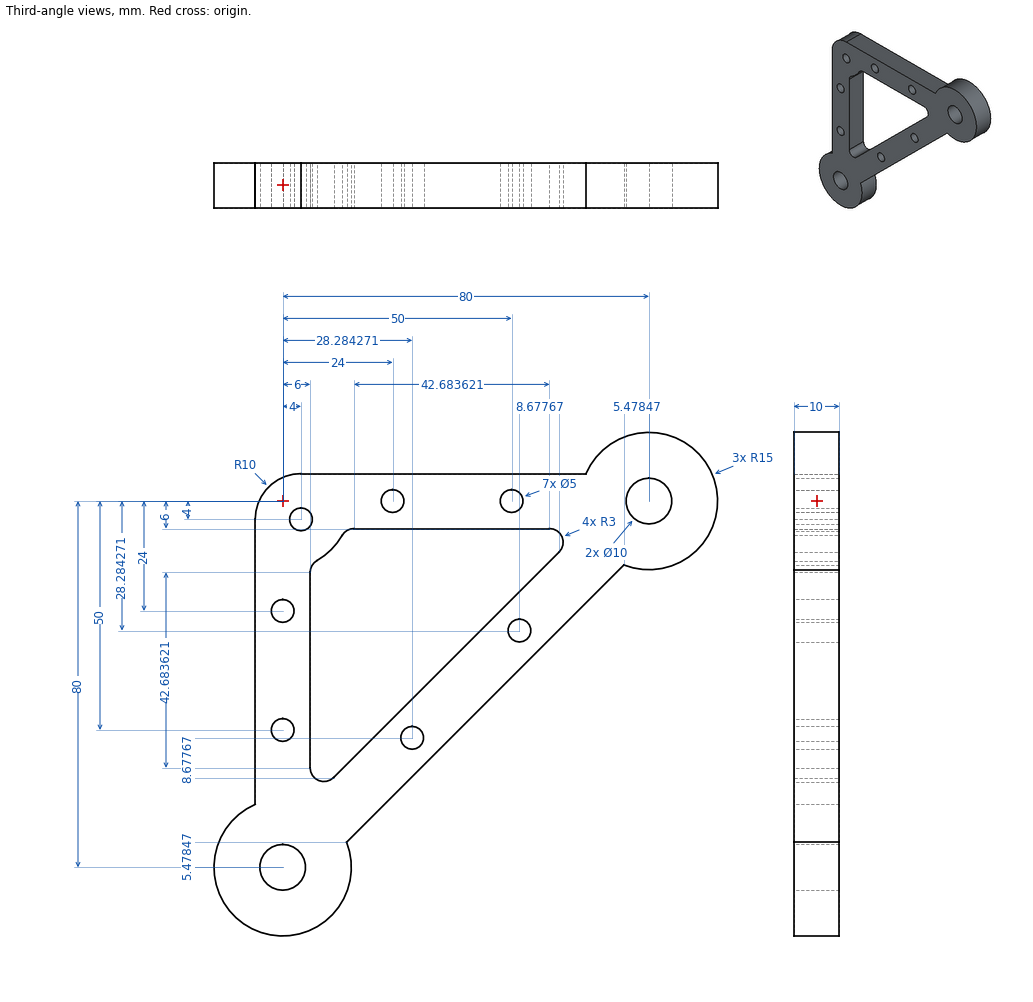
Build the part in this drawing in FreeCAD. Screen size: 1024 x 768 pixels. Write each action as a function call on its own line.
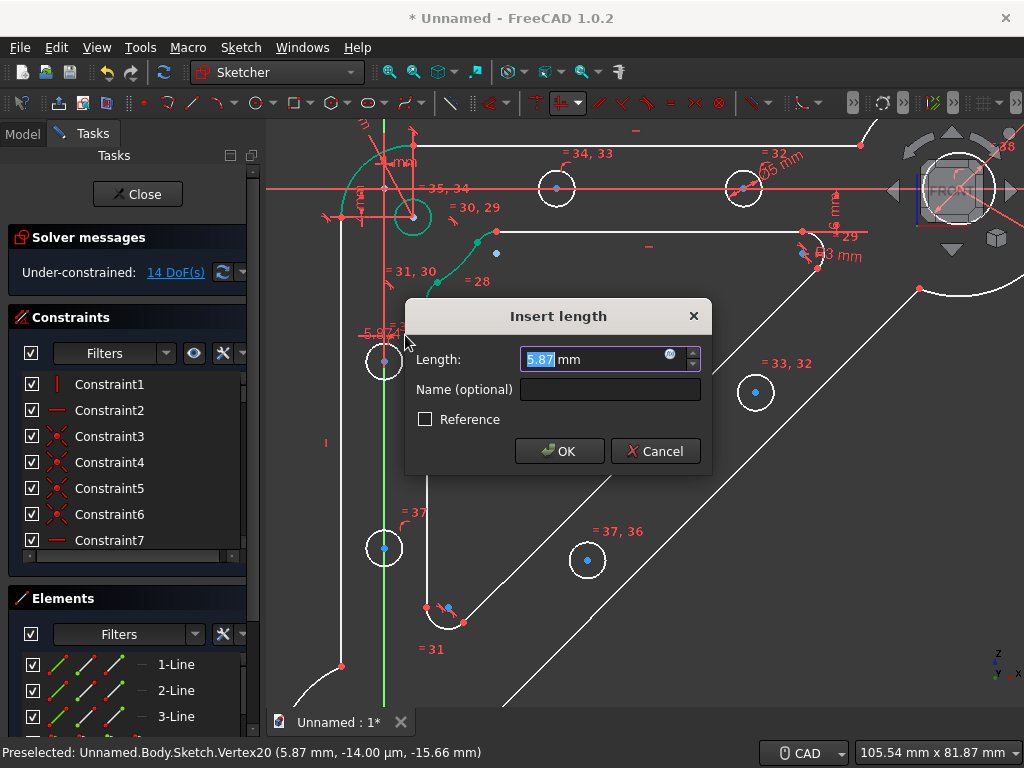
text(6)
key(Return)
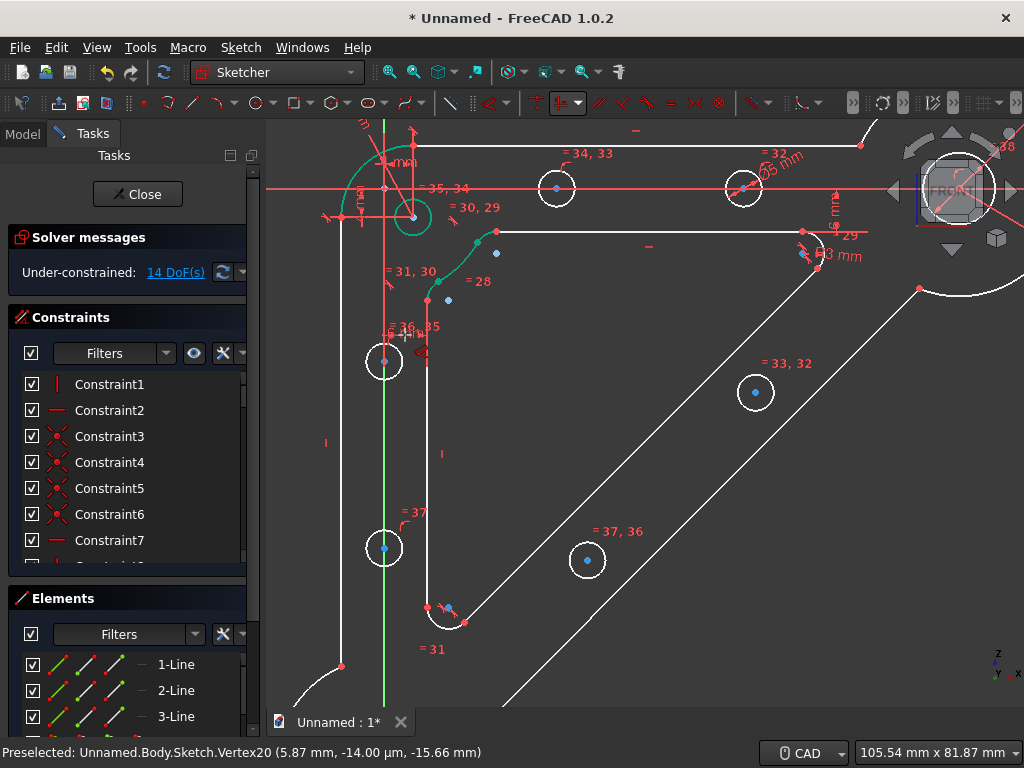
scroll(426, 302, down, 3)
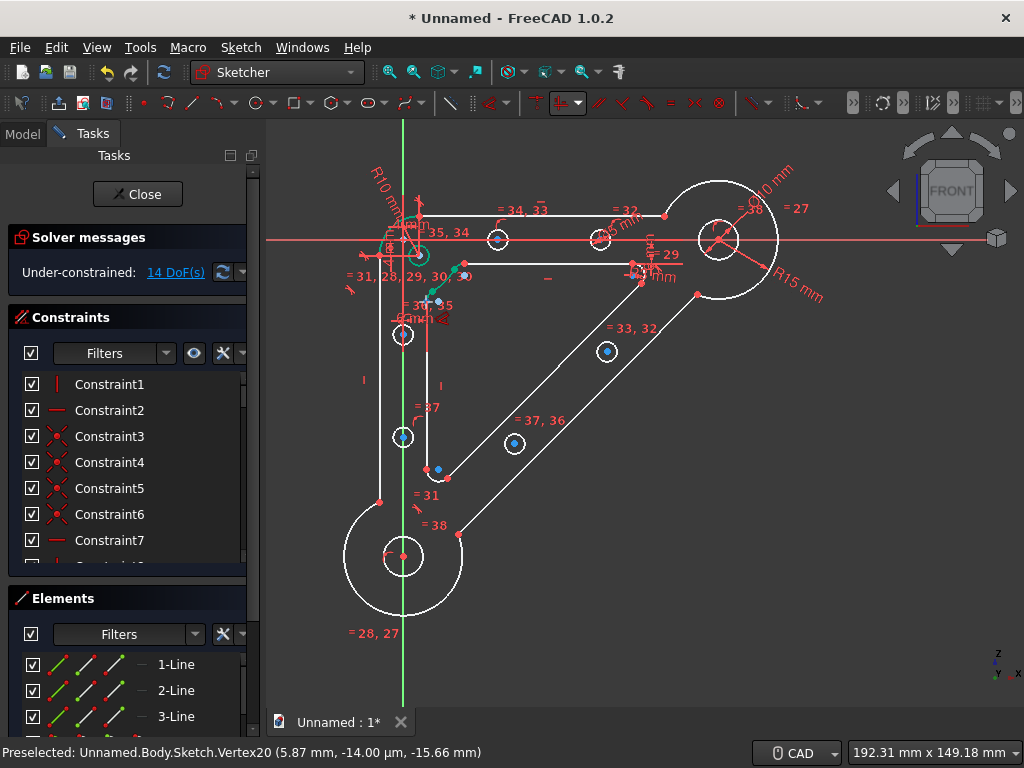
click(719, 240)
click(561, 182)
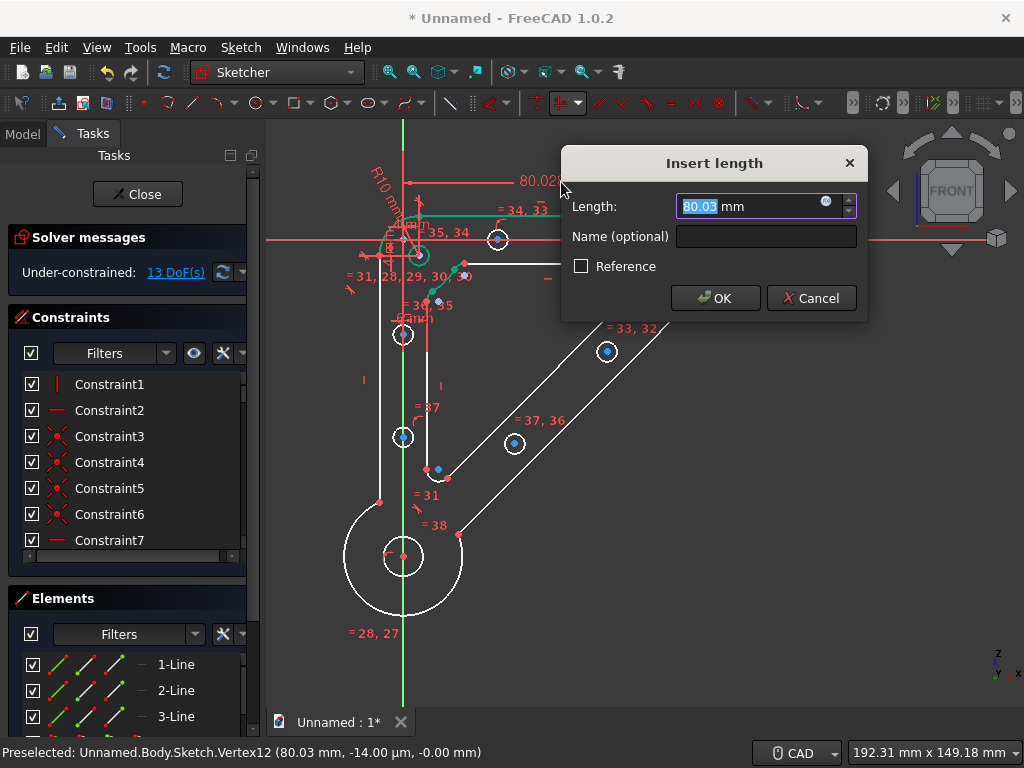
text(80)
key(Return)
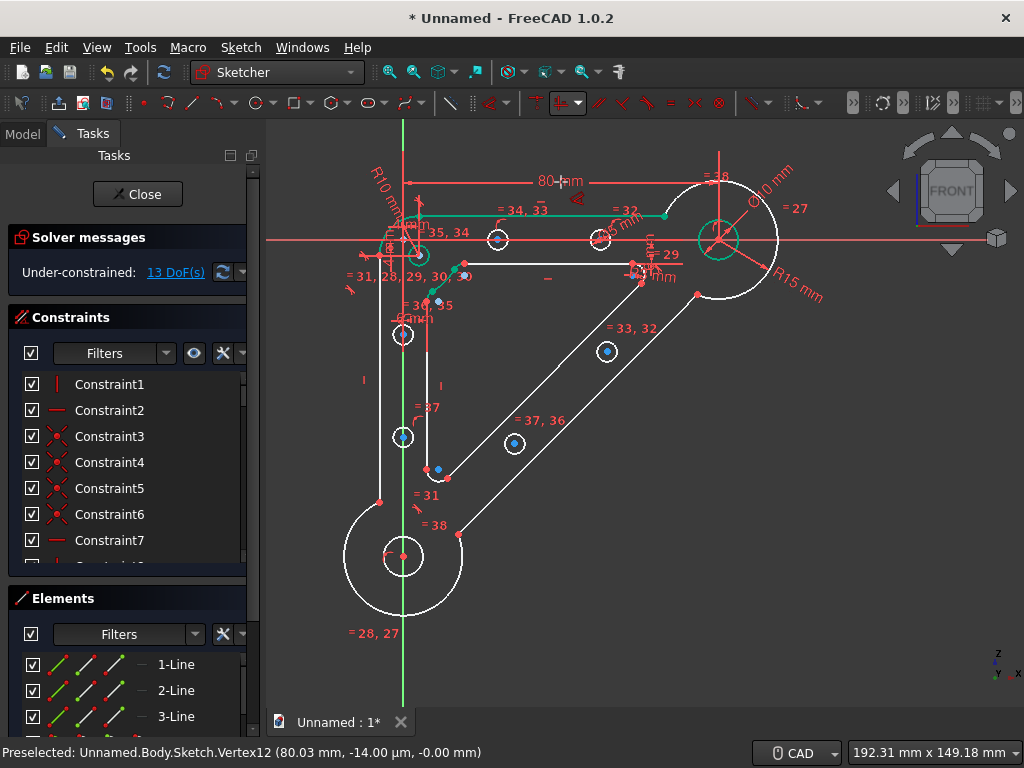
click(600, 240)
click(433, 274)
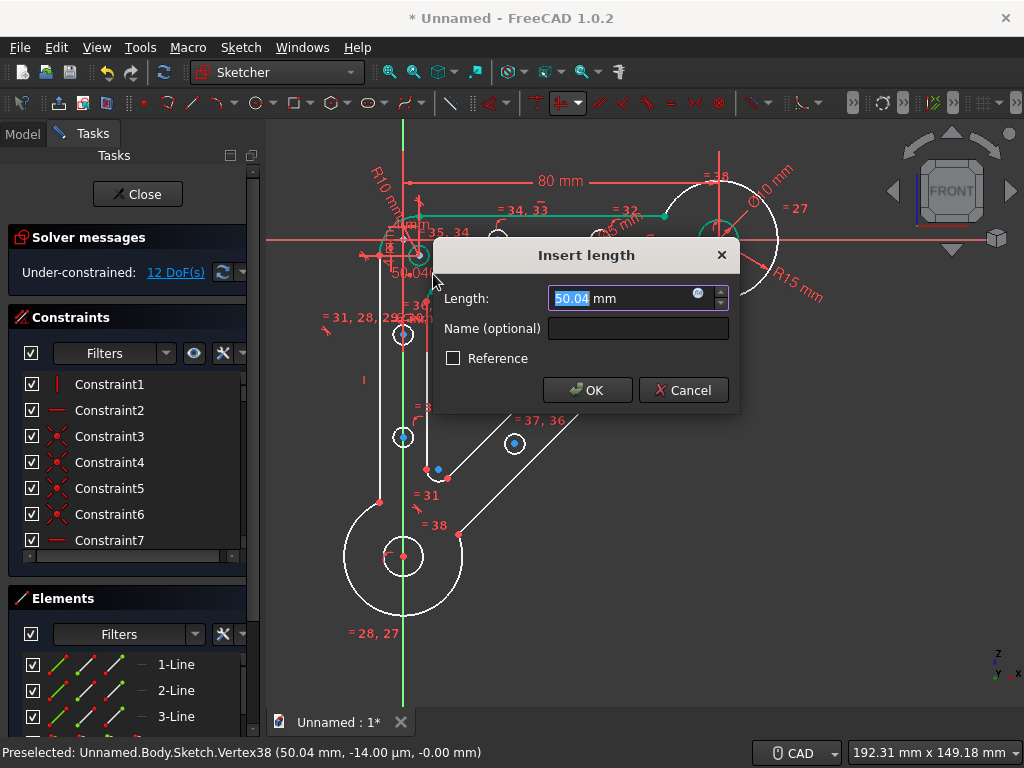
text(50)
key(Return)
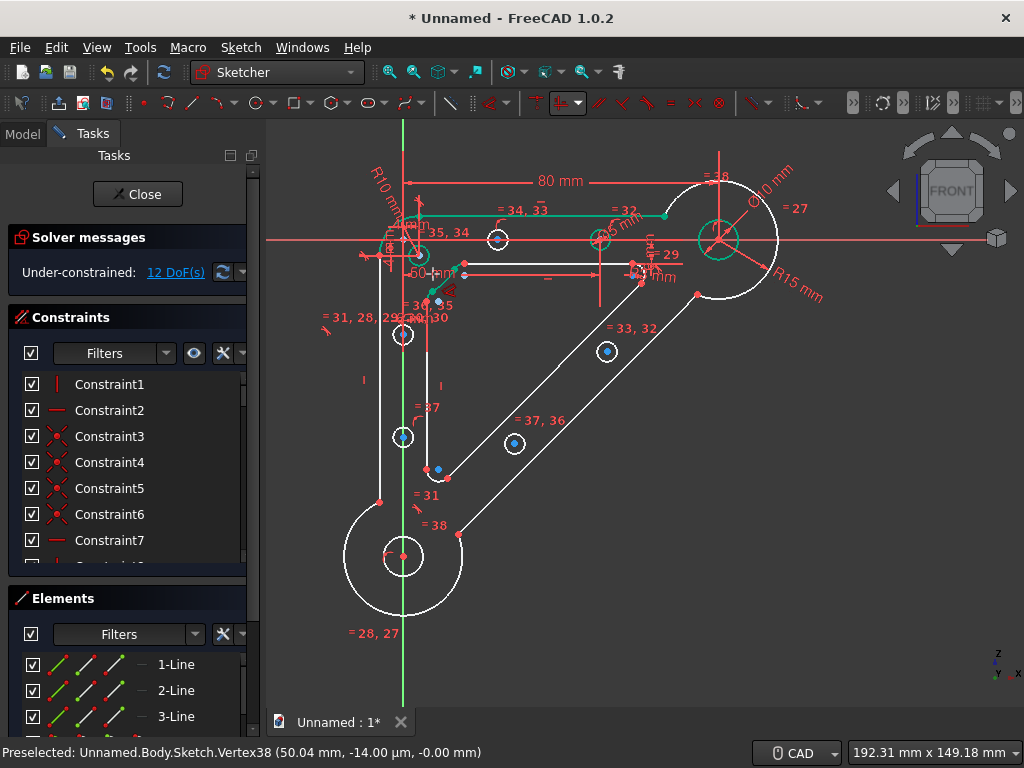
click(498, 240)
click(472, 182)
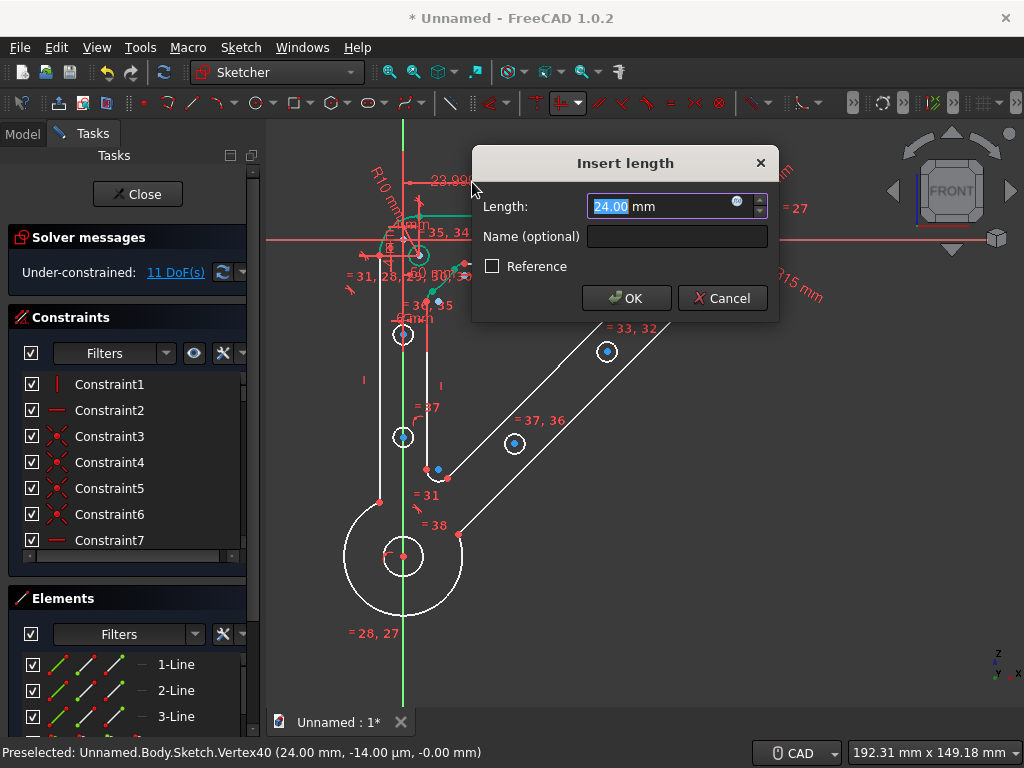
text(24)
key(Return)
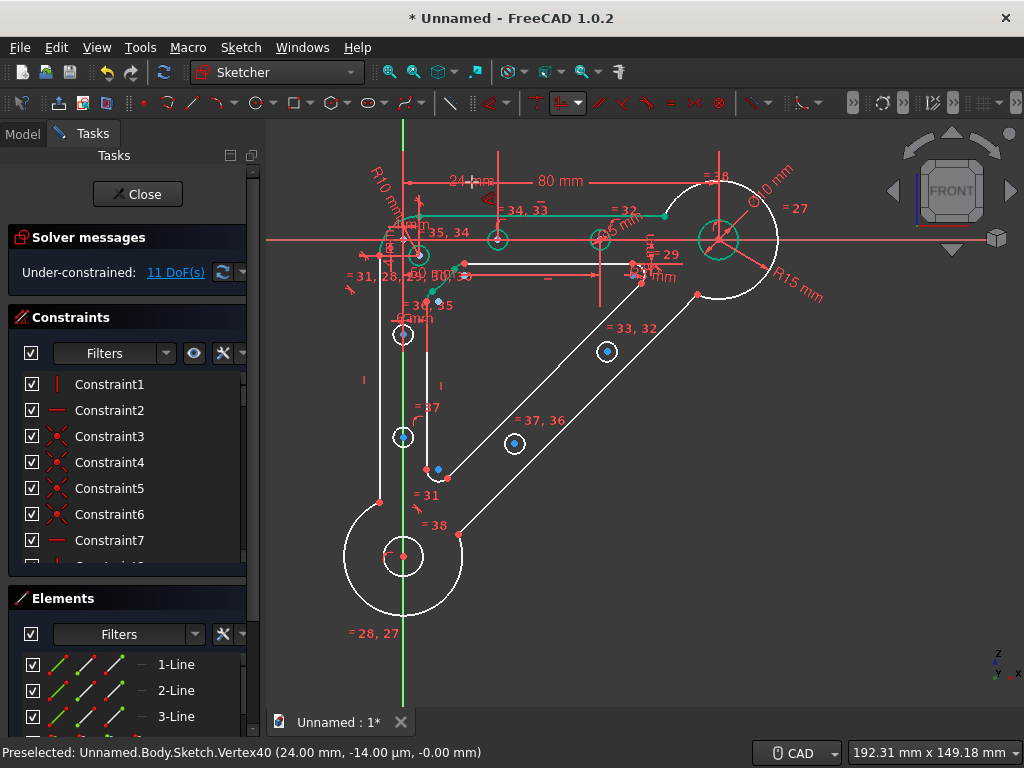
click(403, 335)
click(345, 287)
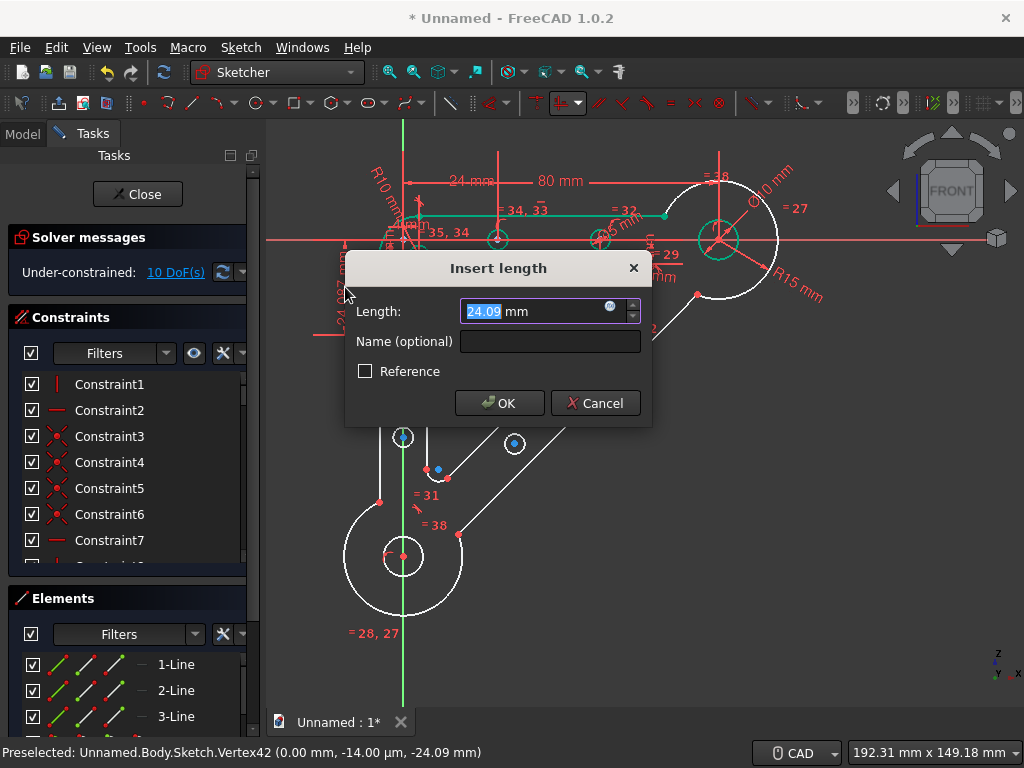
text(24)
key(Return)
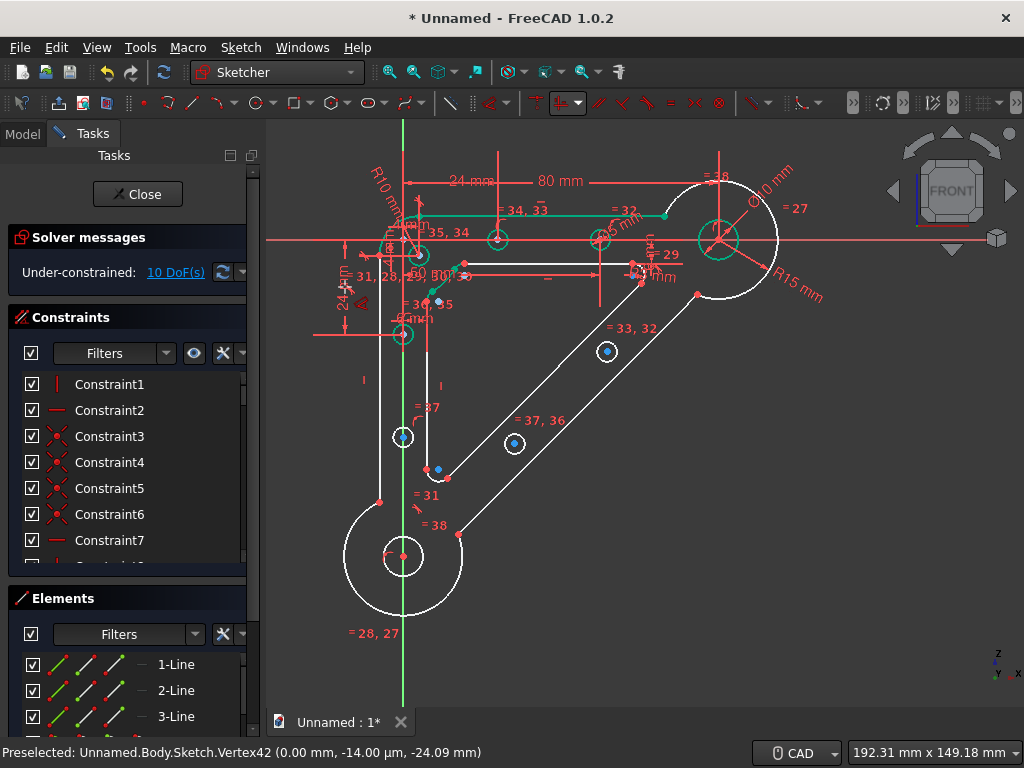
click(403, 437)
click(345, 384)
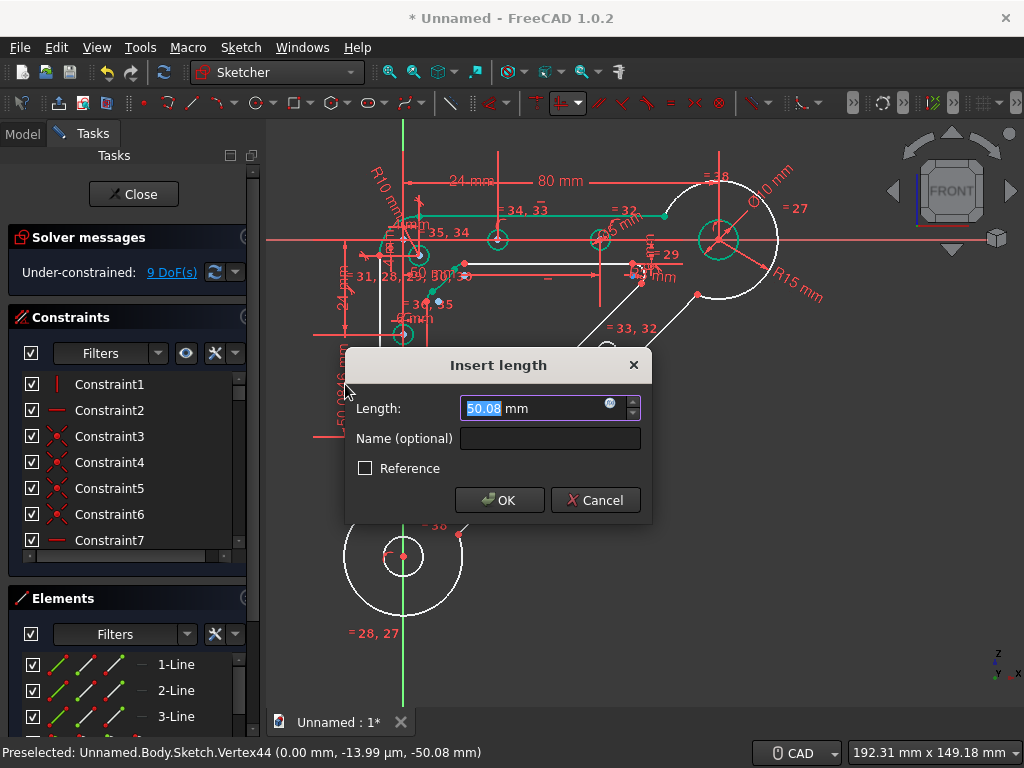
text(50)
key(Return)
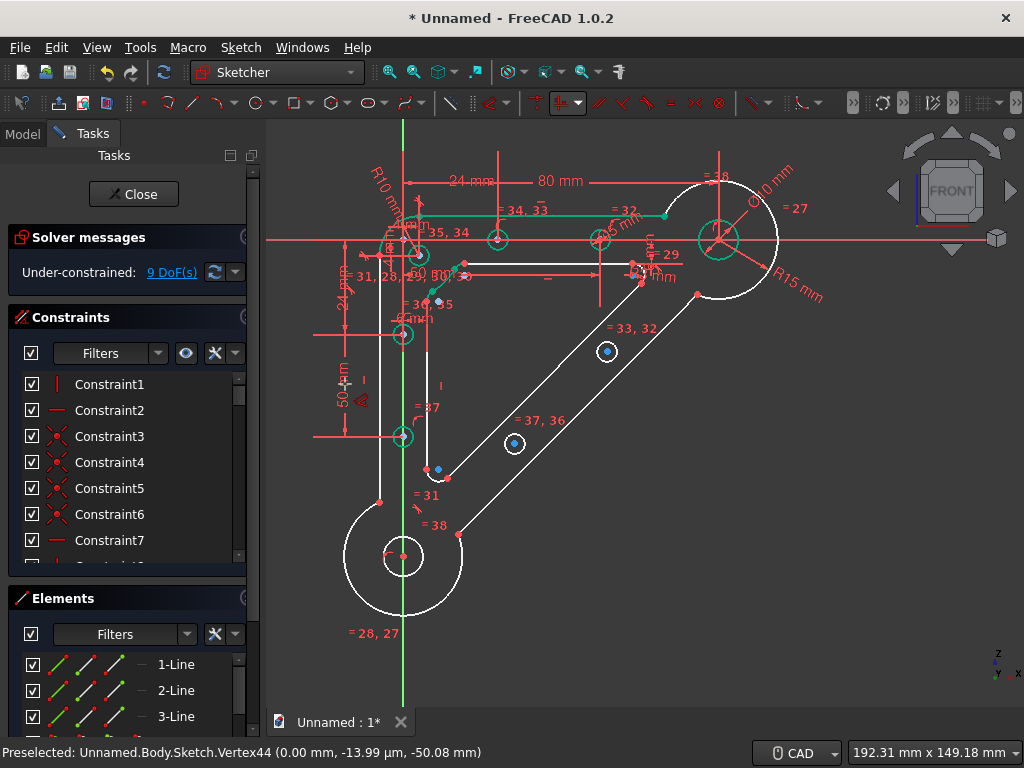
click(403, 557)
click(437, 509)